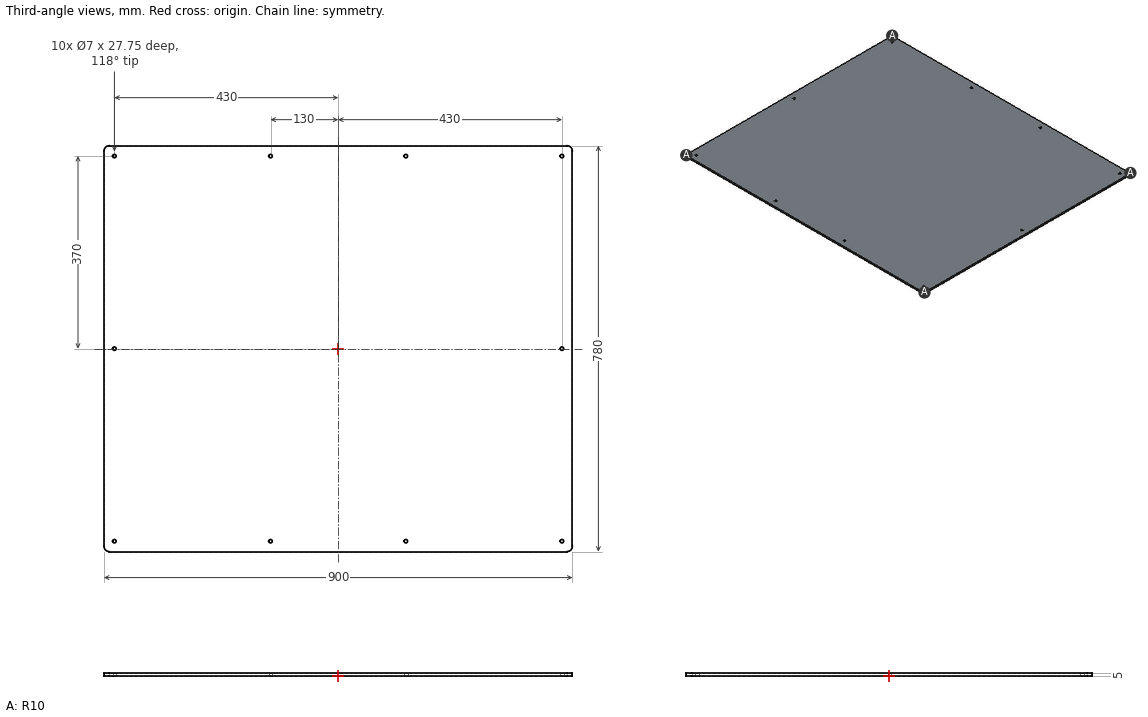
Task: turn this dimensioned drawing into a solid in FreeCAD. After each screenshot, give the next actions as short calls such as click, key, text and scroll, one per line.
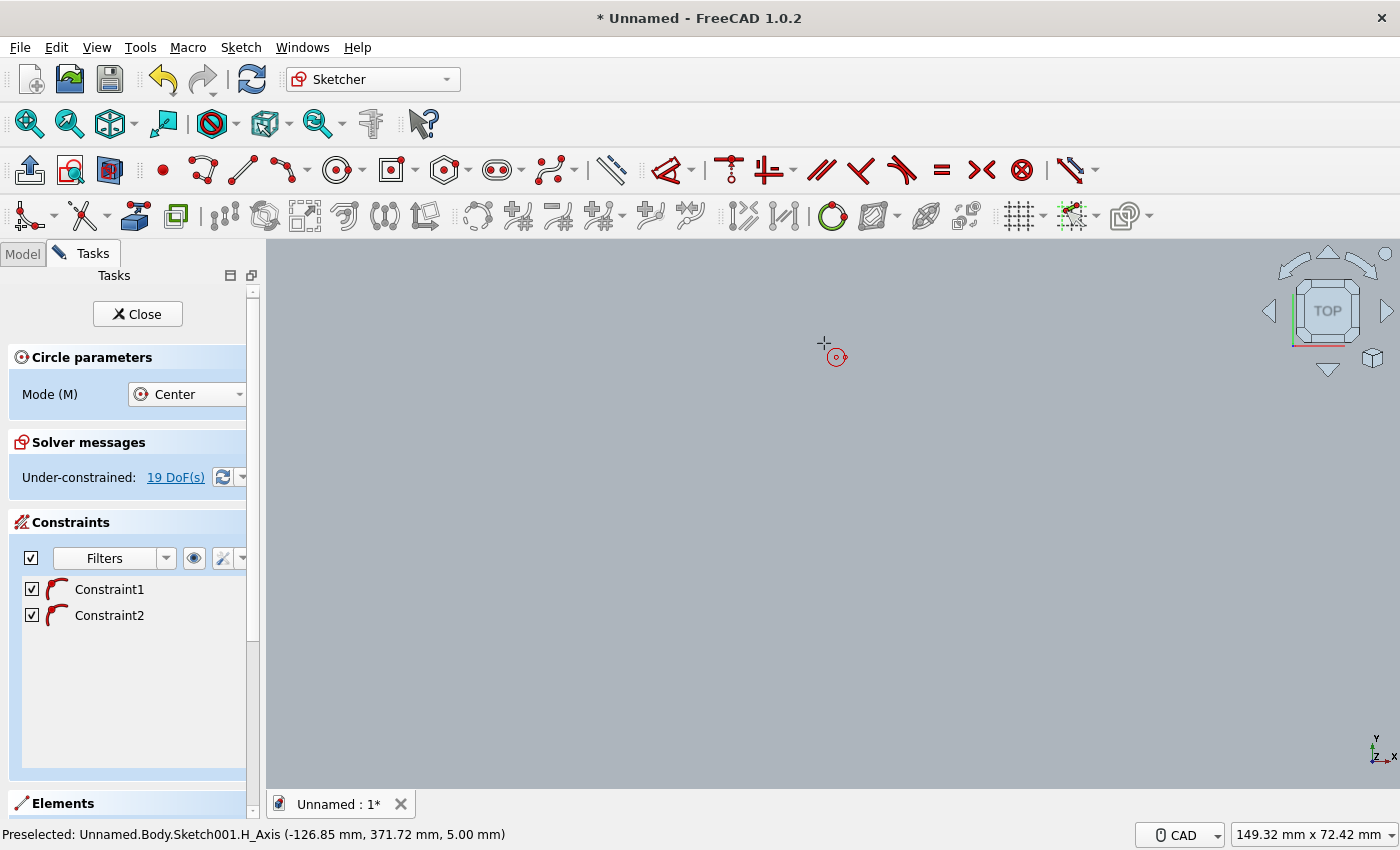
scroll(825, 343, down, 14)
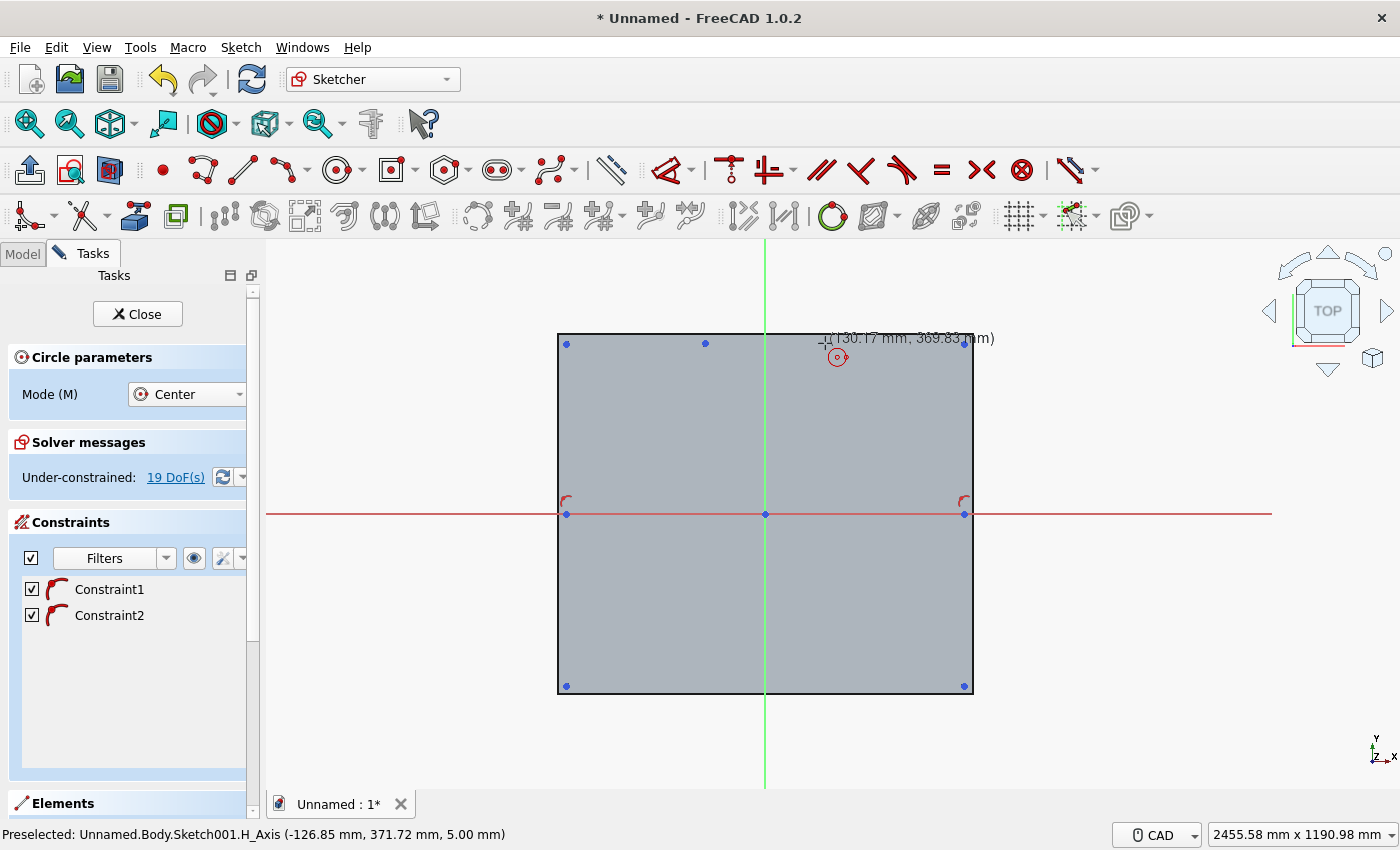
click(825, 343)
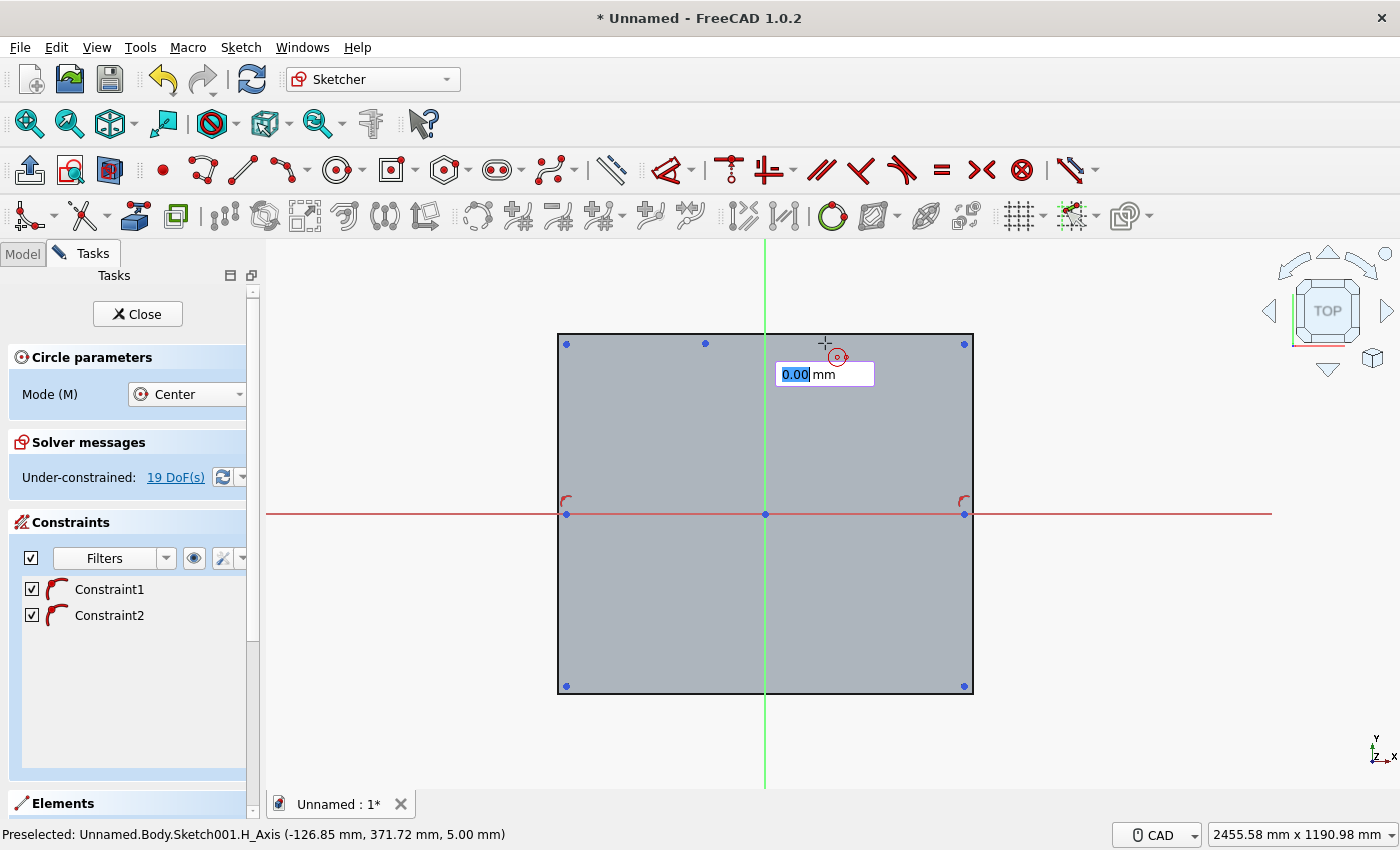
scroll(827, 342, up, 12)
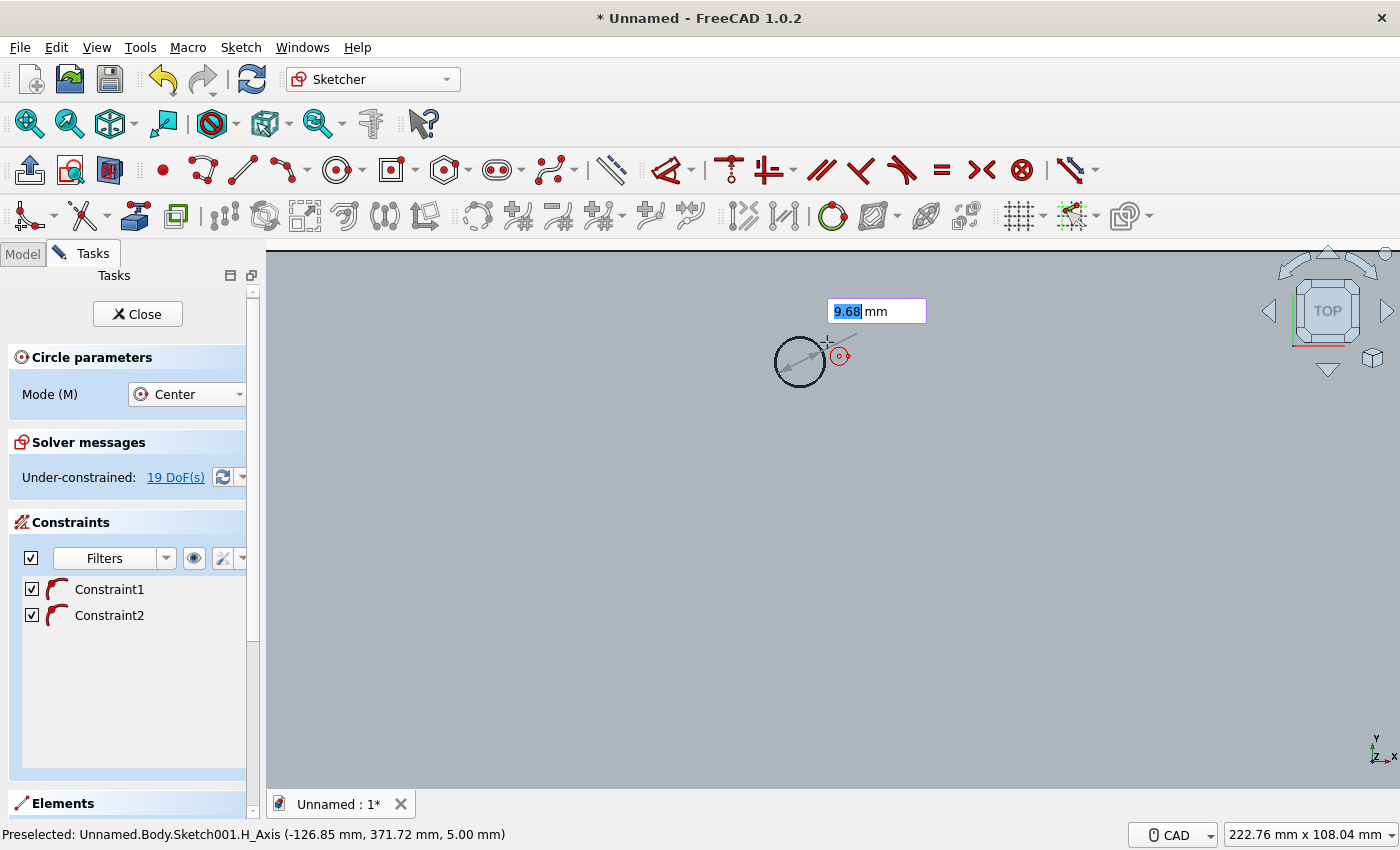
click(817, 340)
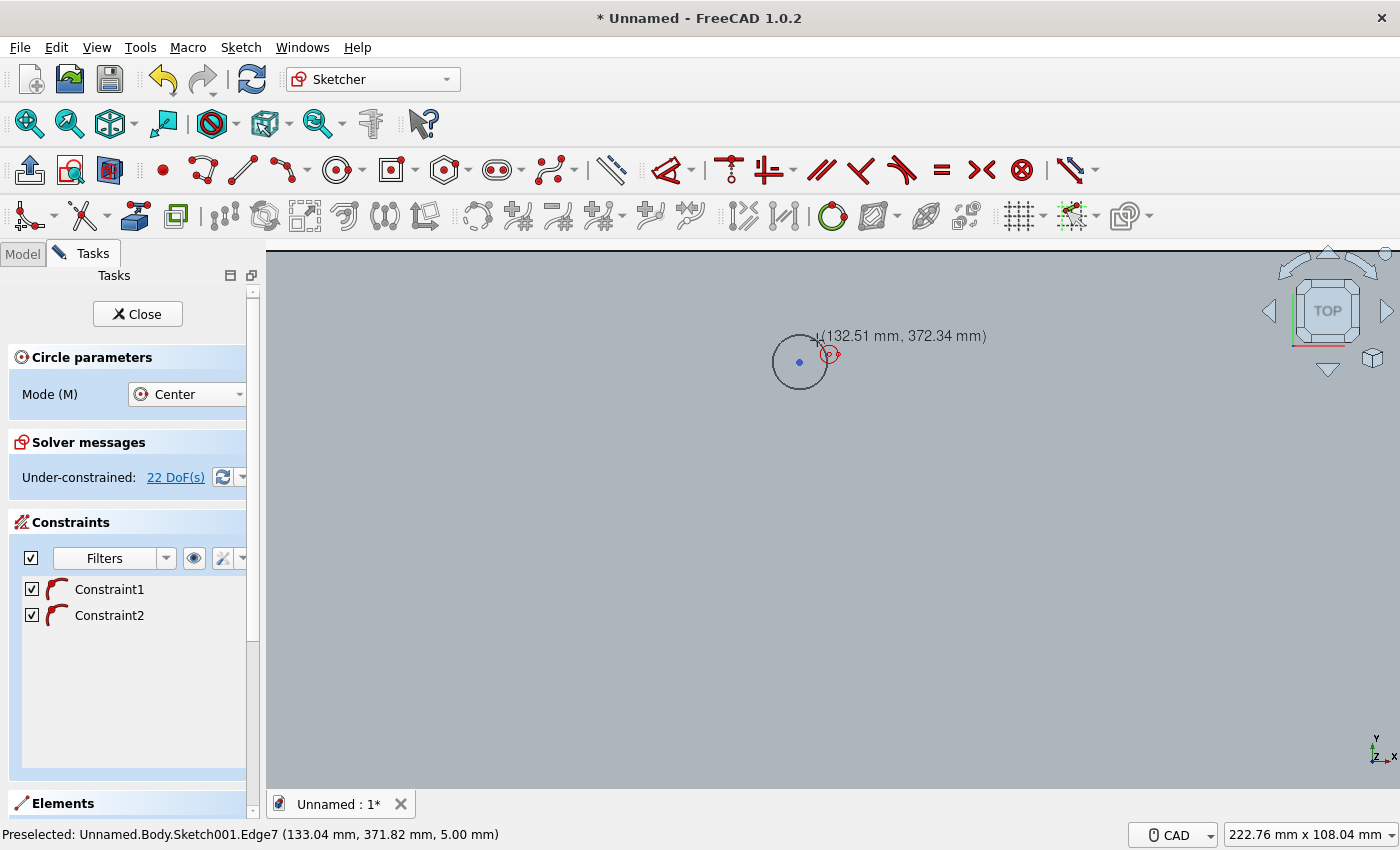
scroll(827, 342, down, 12)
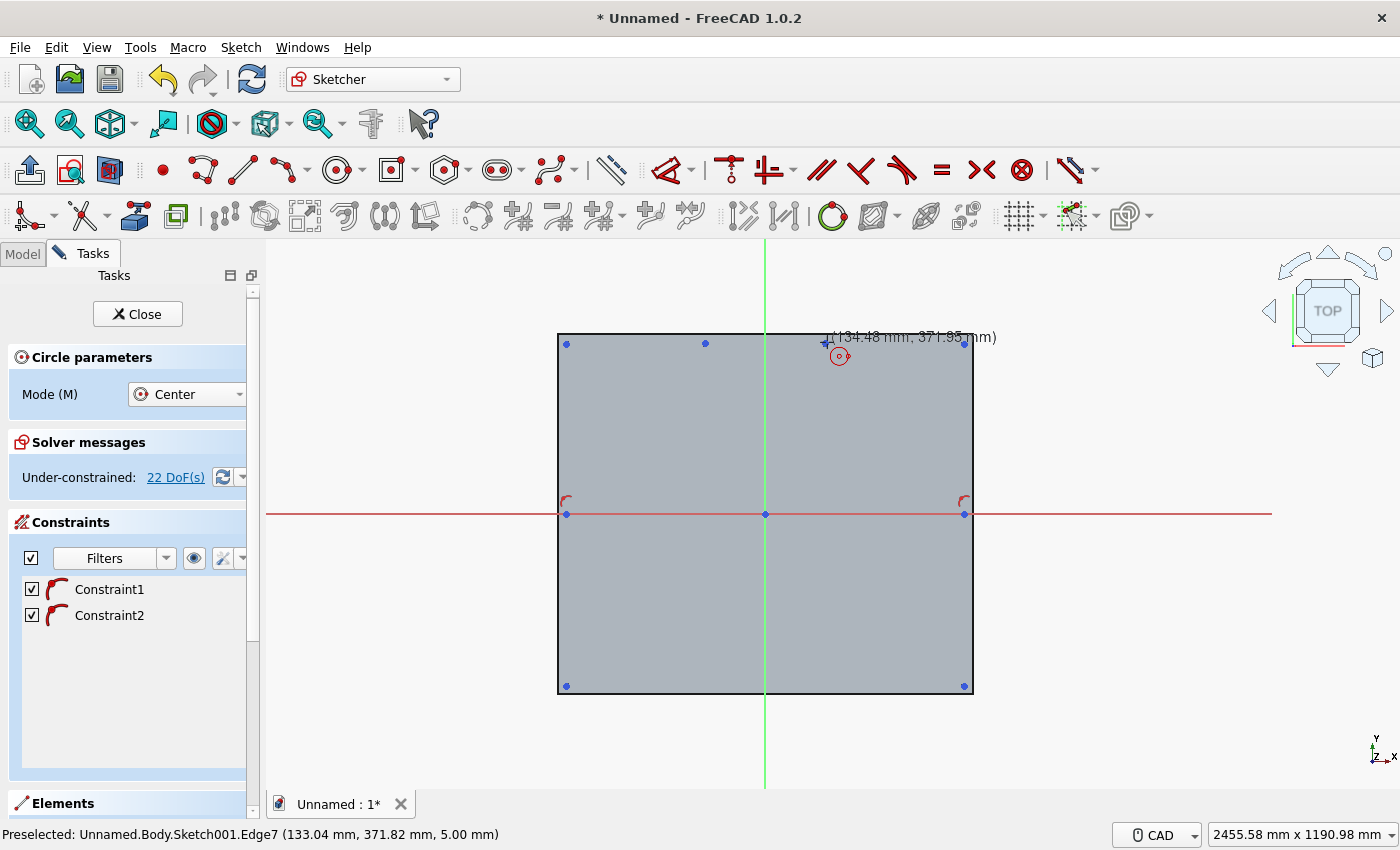
scroll(705, 685, up, 14)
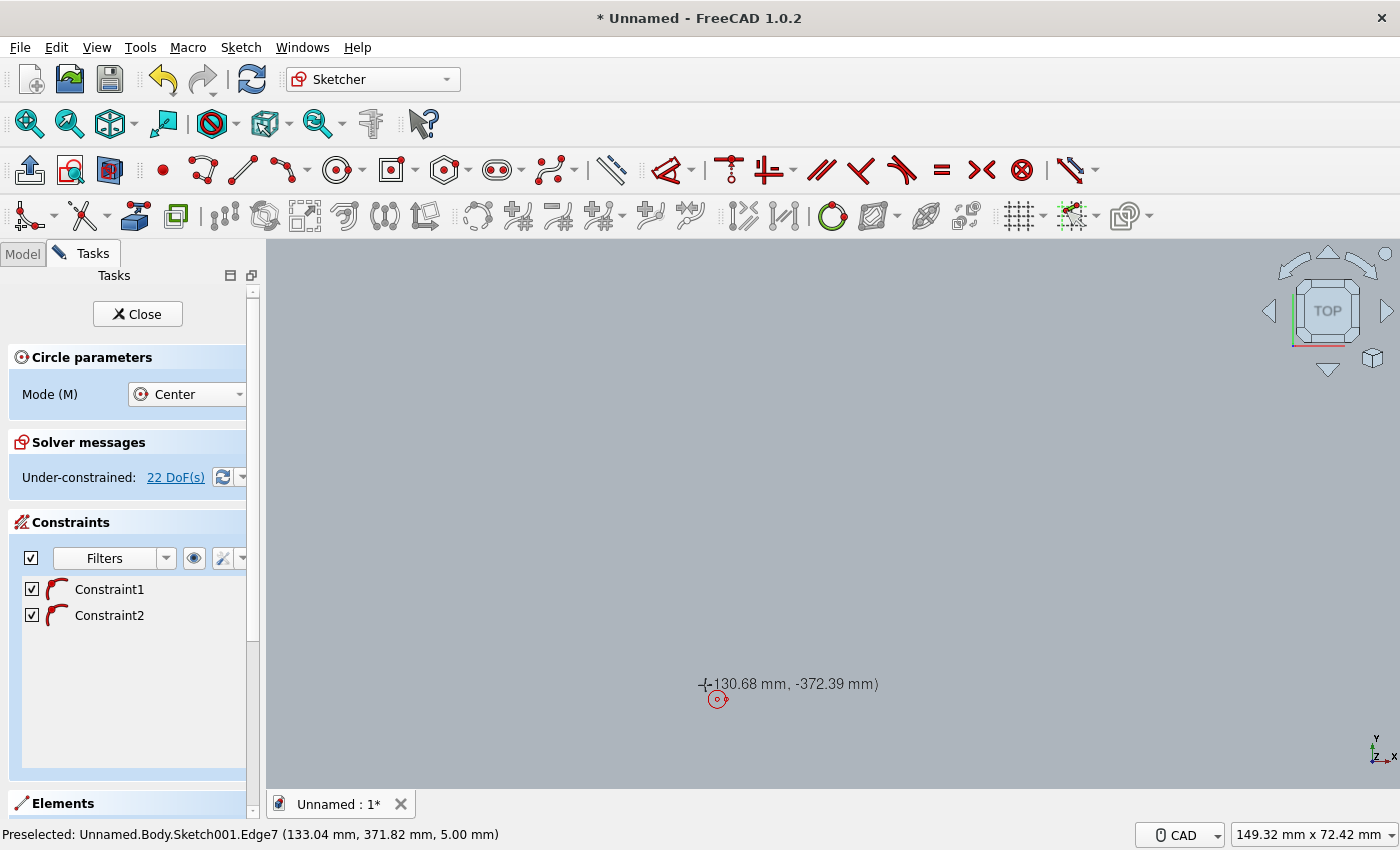
scroll(704, 686, down, 14)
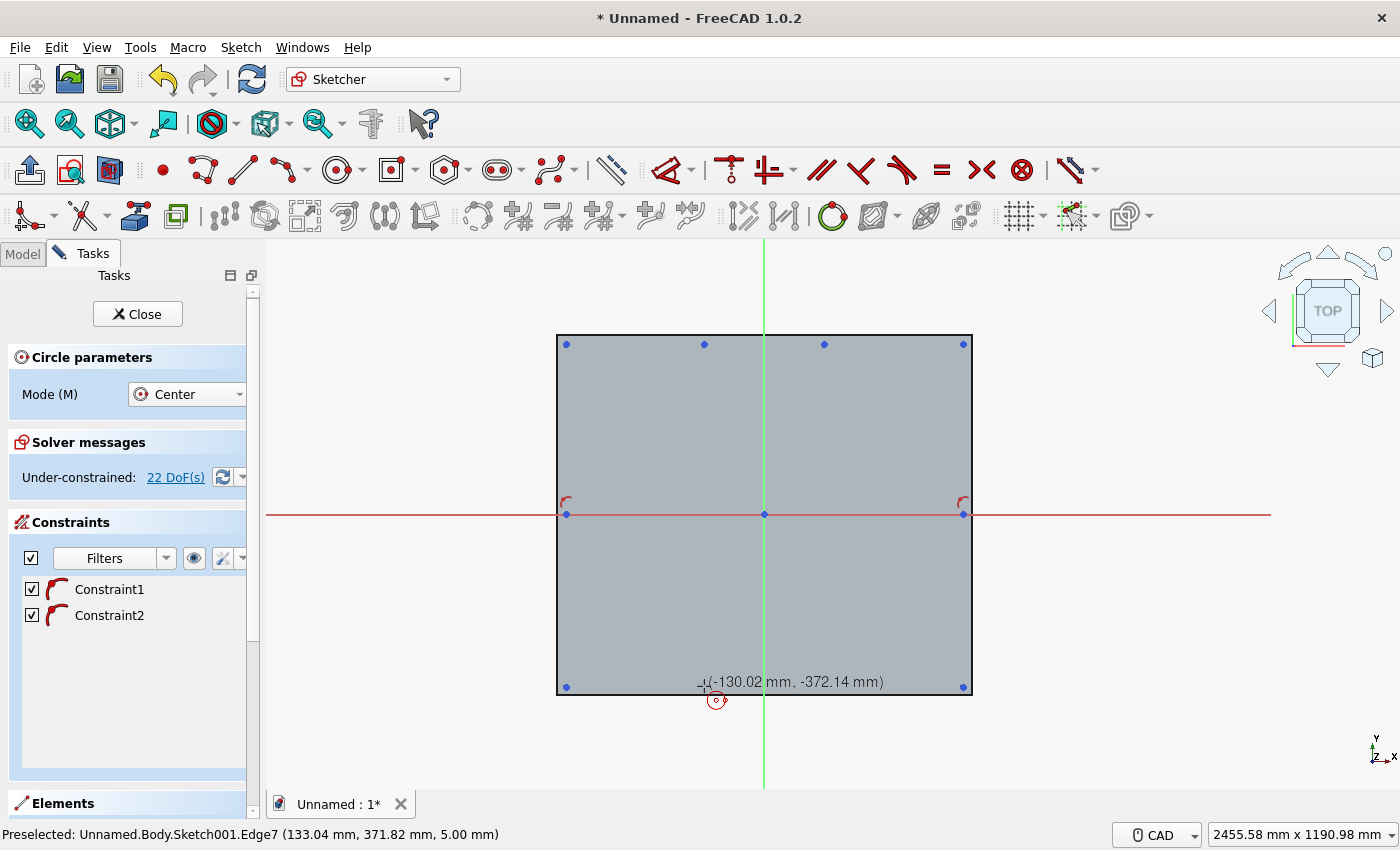
click(704, 686)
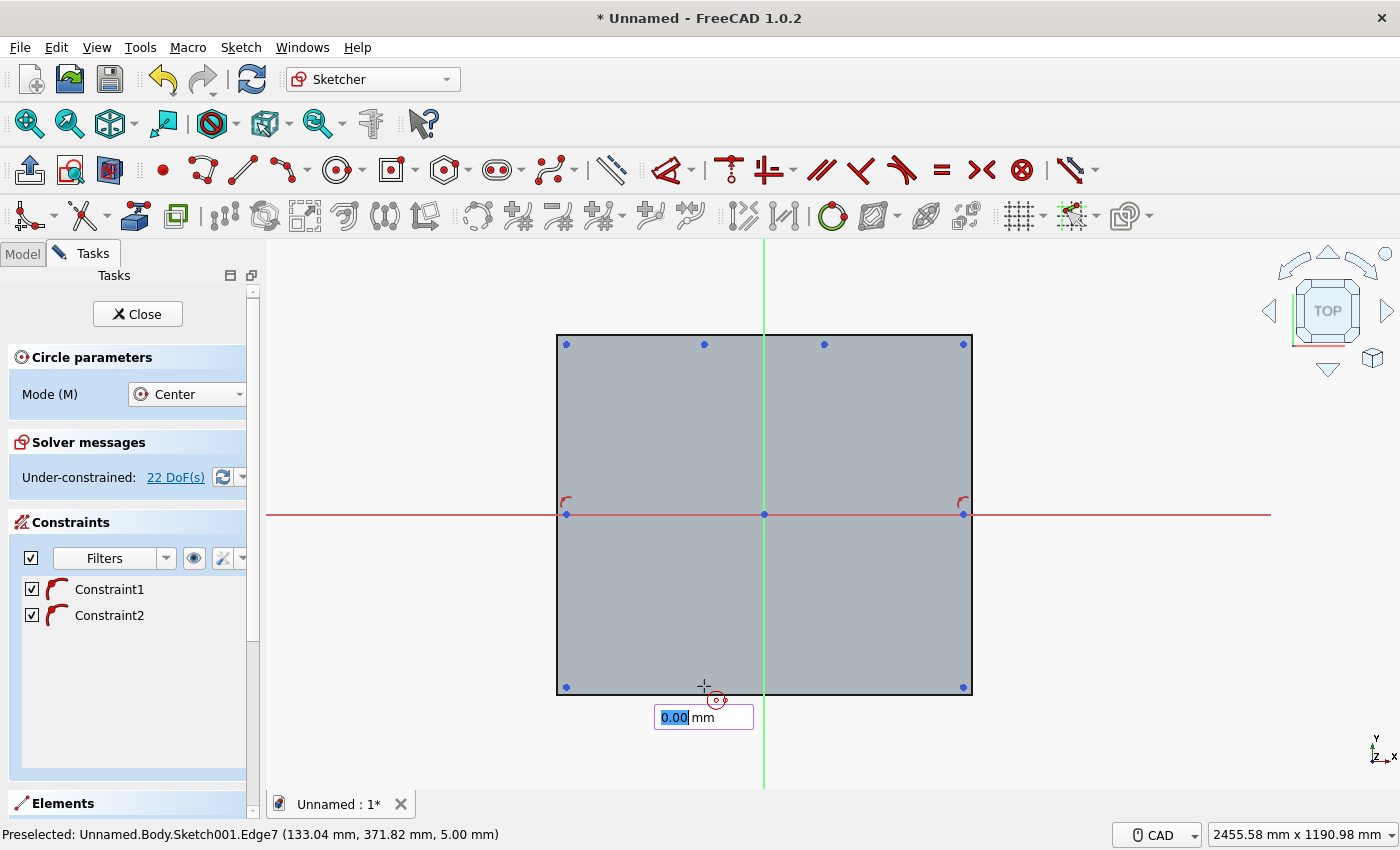
scroll(706, 685, up, 12)